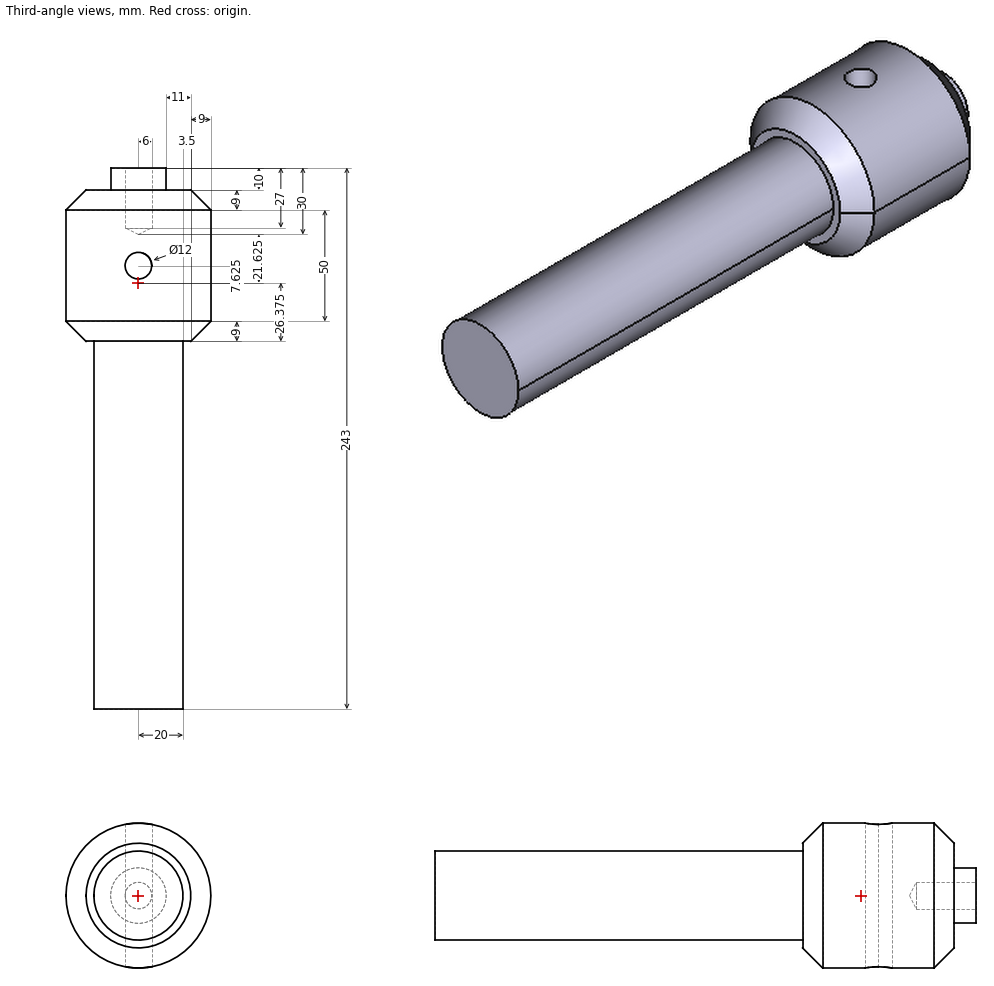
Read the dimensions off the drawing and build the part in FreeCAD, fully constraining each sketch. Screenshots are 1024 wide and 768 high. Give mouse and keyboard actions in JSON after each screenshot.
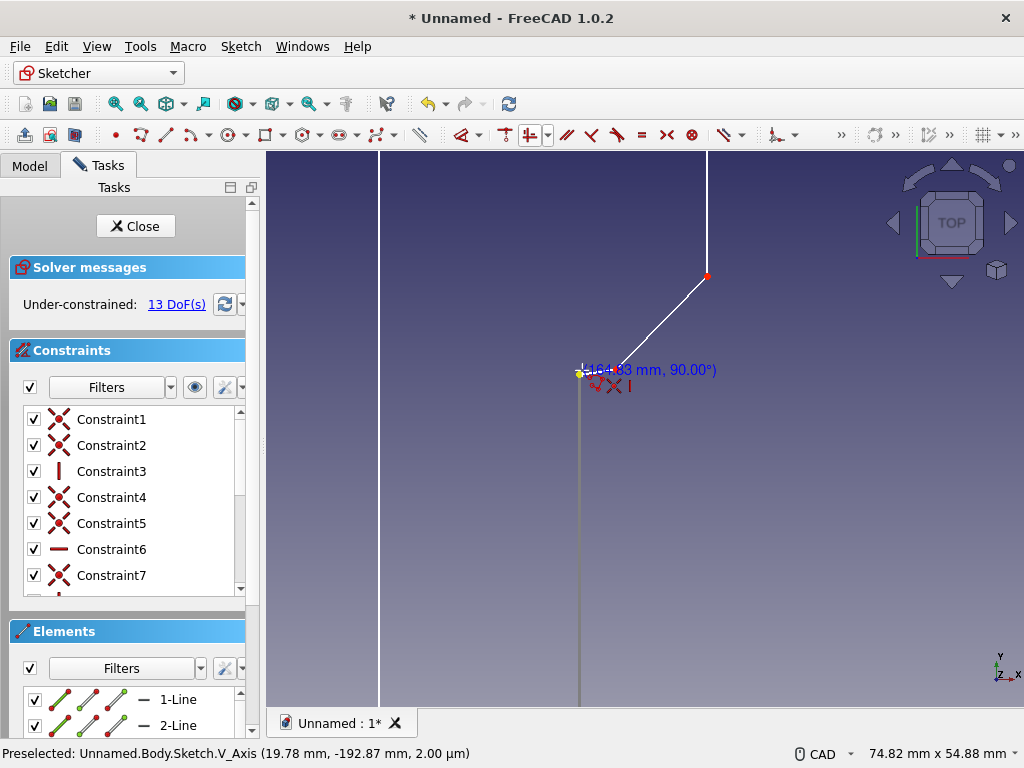
{"action": "left_click", "coordinate": [579, 375]}
{"action": "key", "text": "Escape"}
{"action": "key", "text": "Escape"}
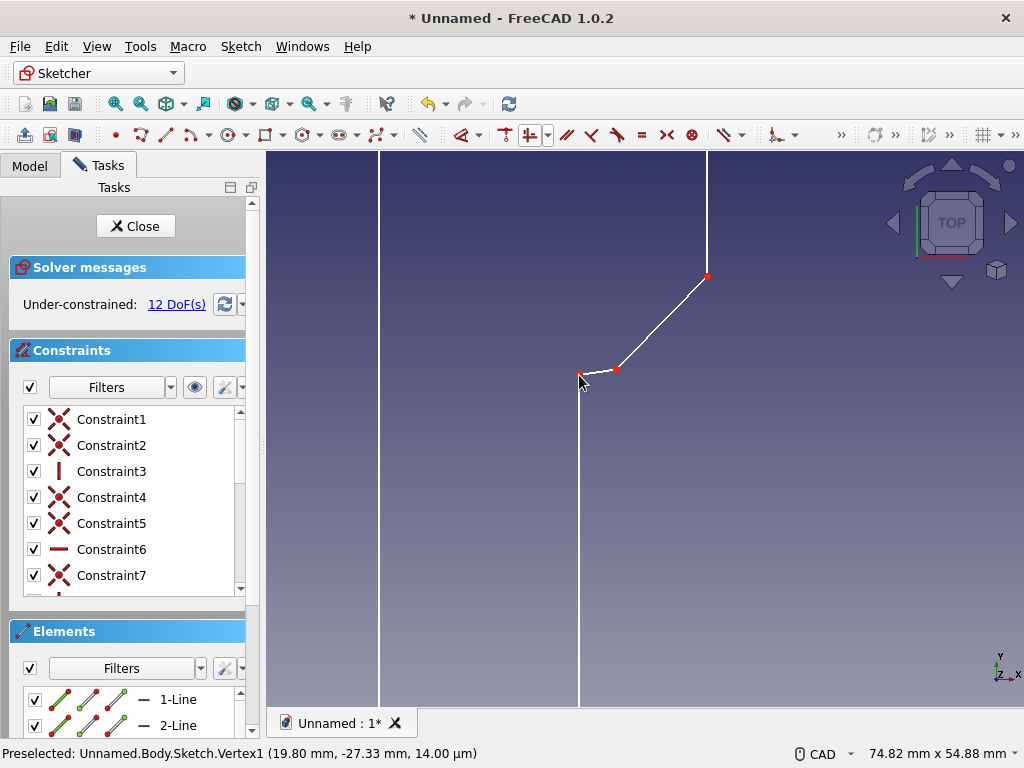
{"action": "scroll", "coordinate": [590, 373], "scroll_direction": "up", "scroll_amount": 2}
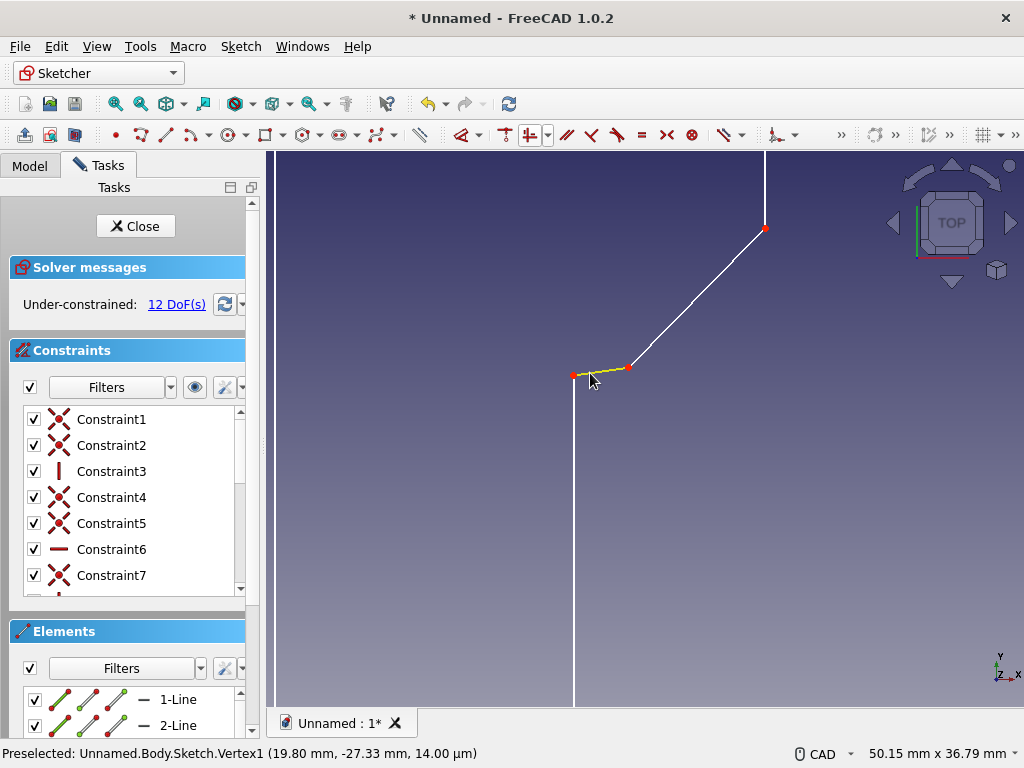
{"action": "left_click", "coordinate": [590, 373]}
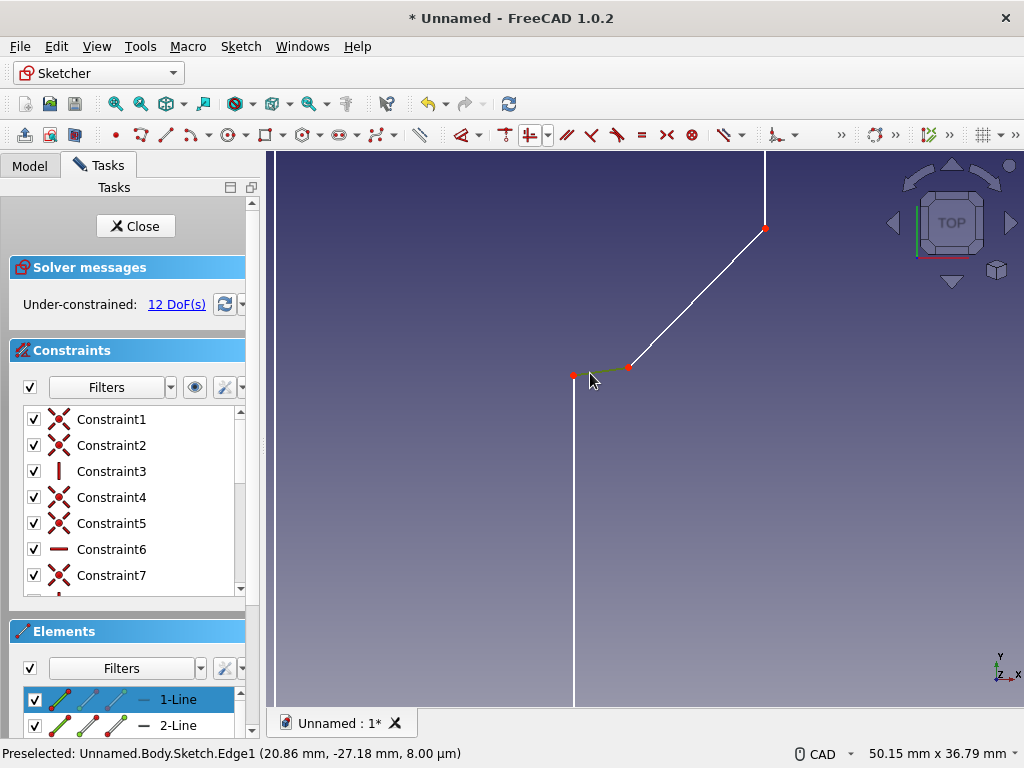
{"action": "key", "text": "h"}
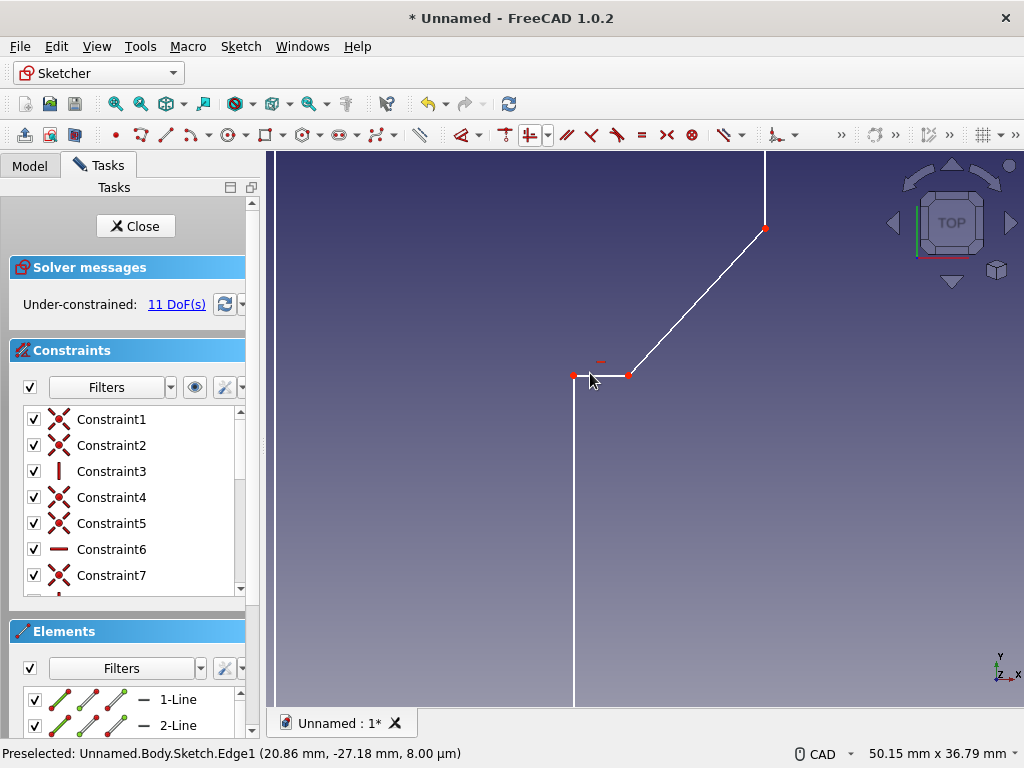
{"action": "key", "text": "d"}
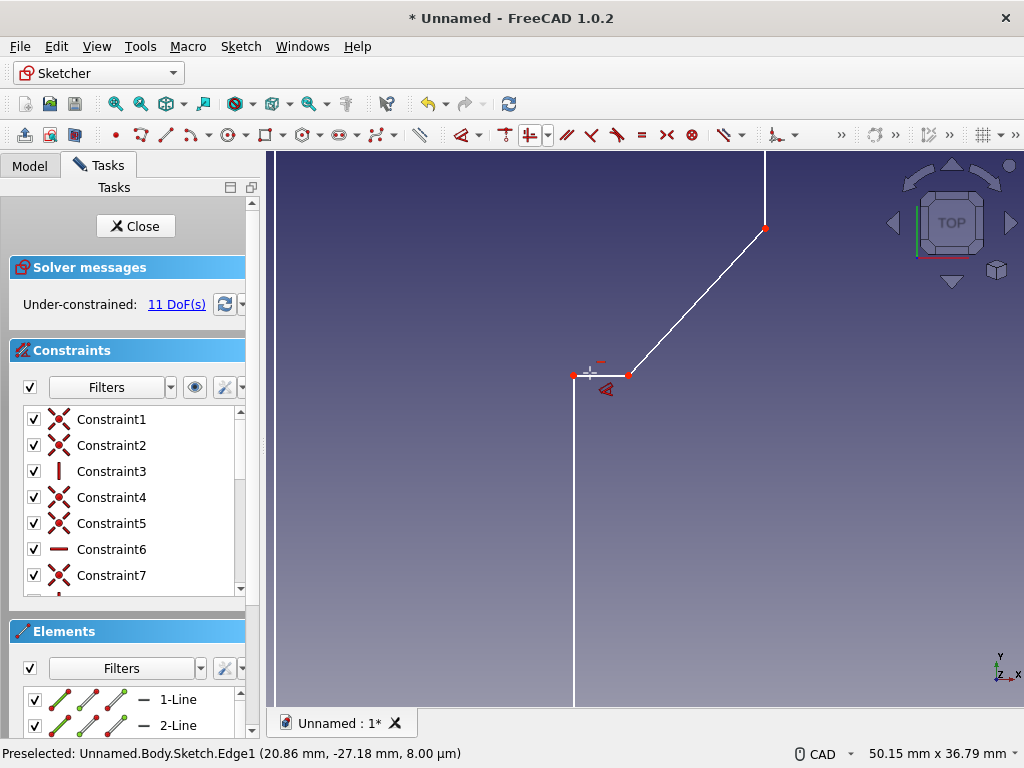
{"action": "scroll", "coordinate": [582, 370], "scroll_direction": "down", "scroll_amount": 12}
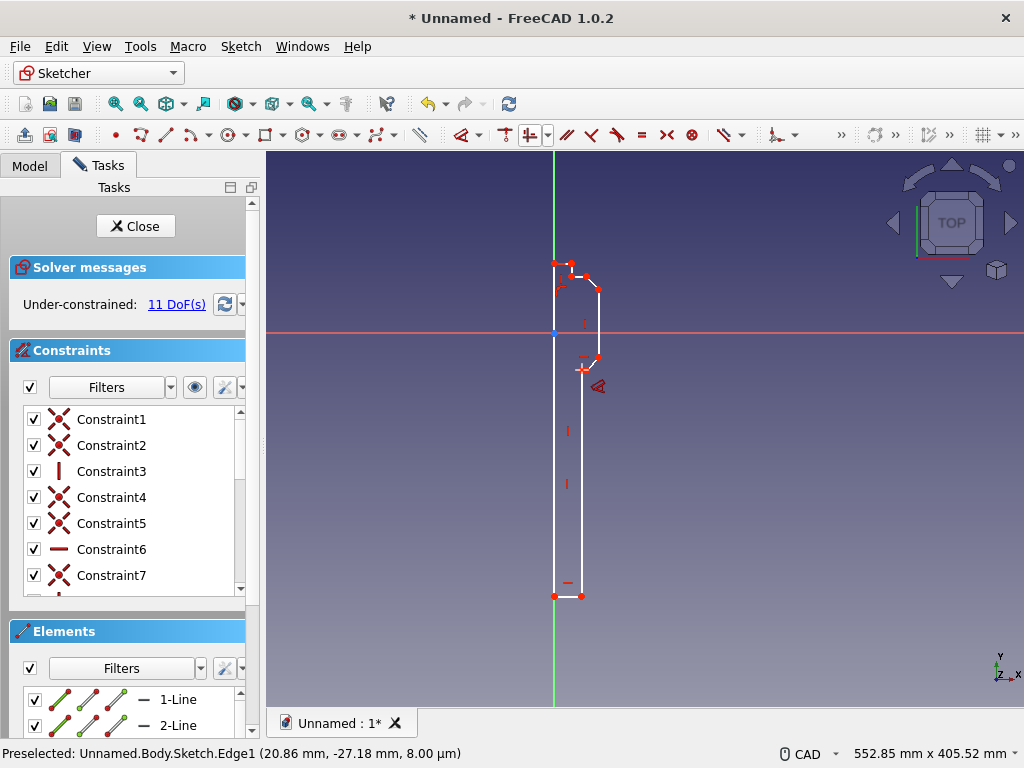
{"action": "scroll", "coordinate": [599, 337], "scroll_direction": "up", "scroll_amount": 7}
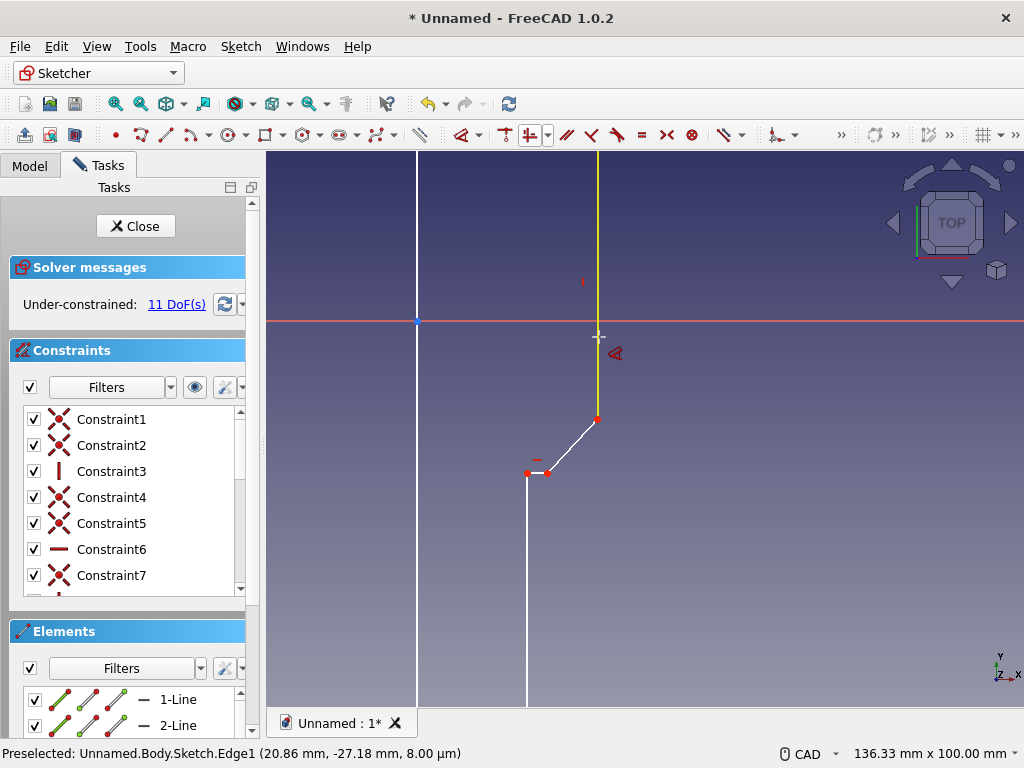
{"action": "left_click", "coordinate": [598, 337]}
{"action": "left_click", "coordinate": [632, 299]}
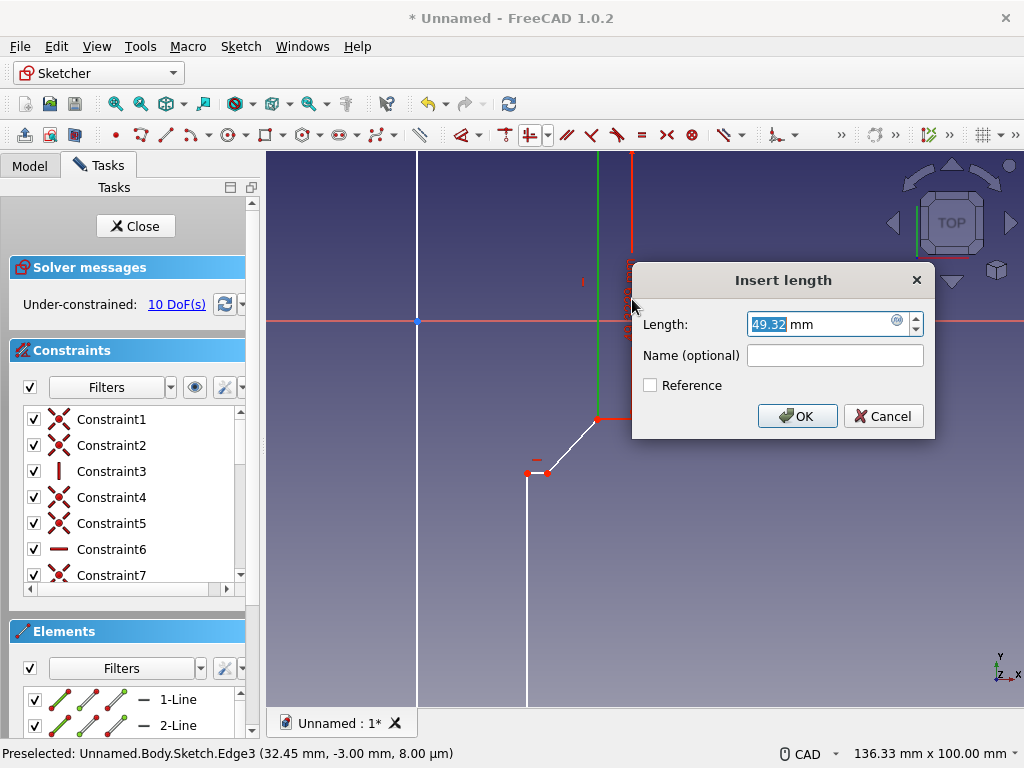
{"action": "type", "text": "50"}
{"action": "key", "text": "Return"}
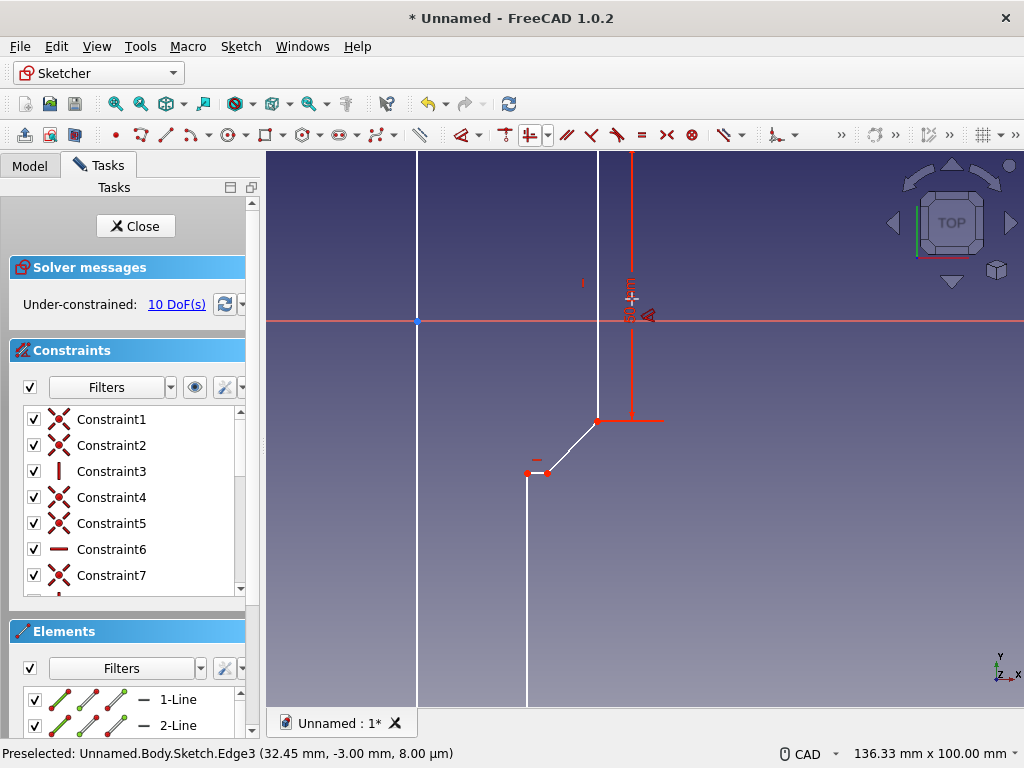
{"action": "scroll", "coordinate": [599, 337], "scroll_direction": "down", "scroll_amount": 7}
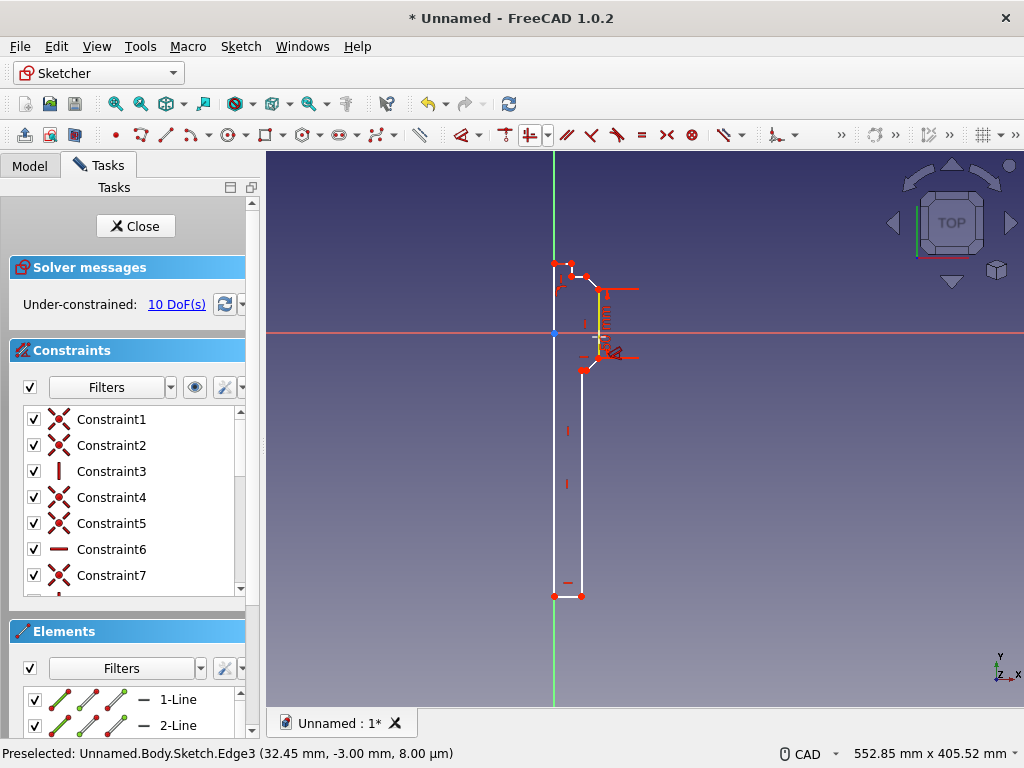
{"action": "scroll", "coordinate": [582, 277], "scroll_direction": "up", "scroll_amount": 6}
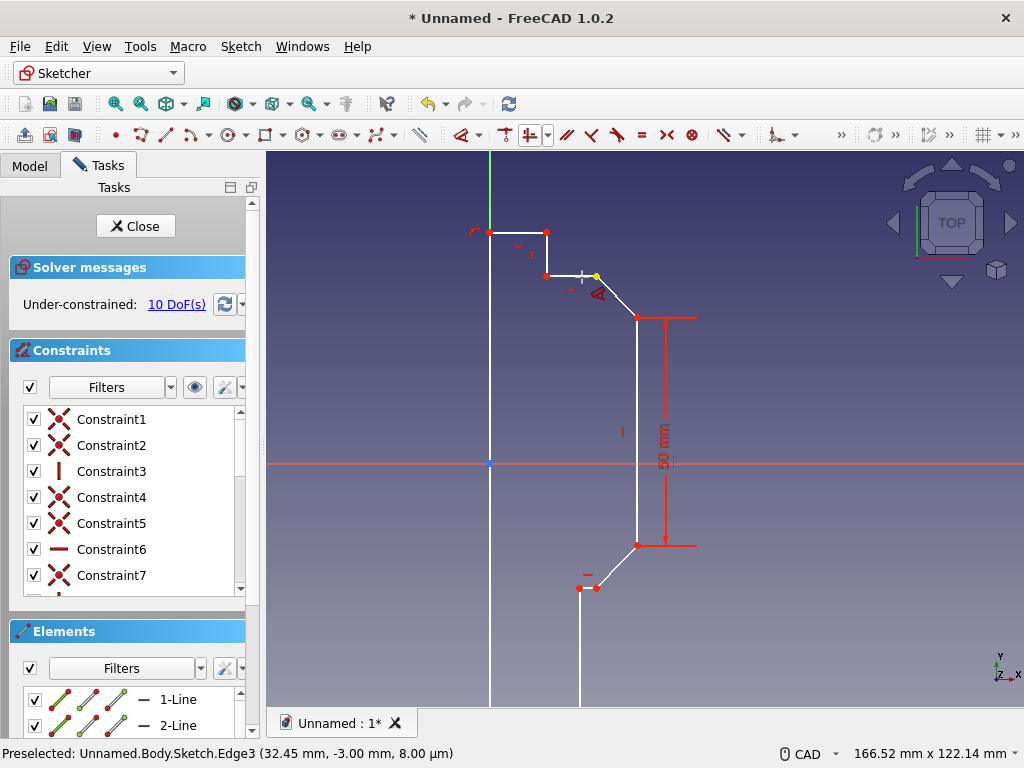
{"action": "left_click", "coordinate": [582, 276]}
{"action": "left_click", "coordinate": [572, 242]}